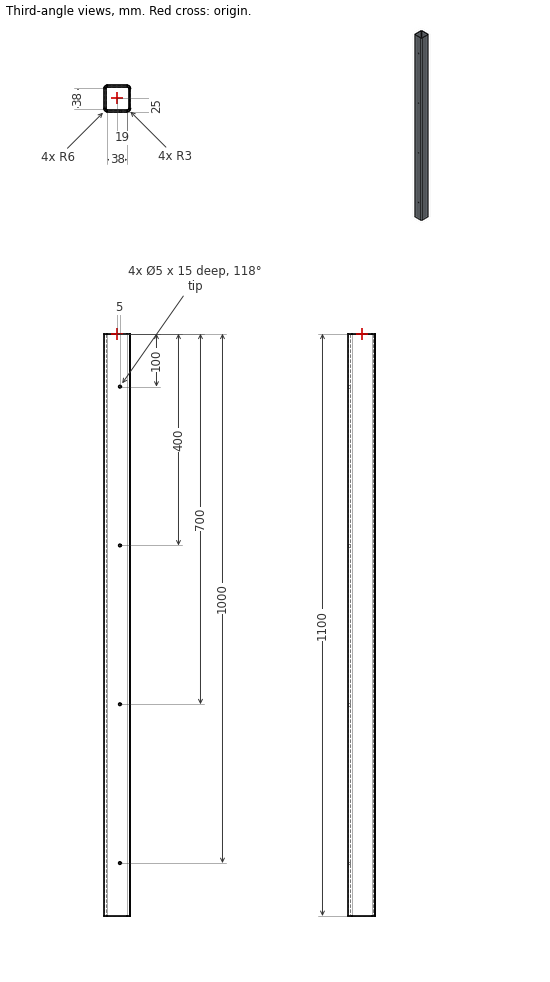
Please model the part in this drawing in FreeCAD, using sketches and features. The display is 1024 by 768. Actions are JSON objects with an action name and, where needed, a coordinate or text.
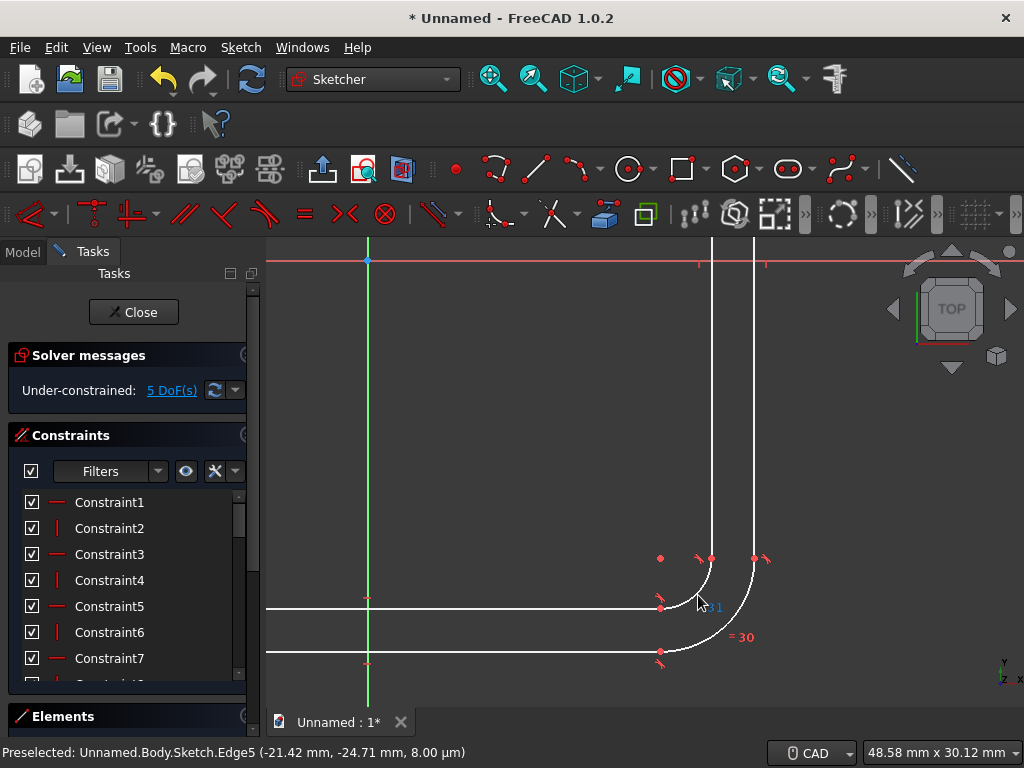
{"action": "left_click", "coordinate": [697, 594]}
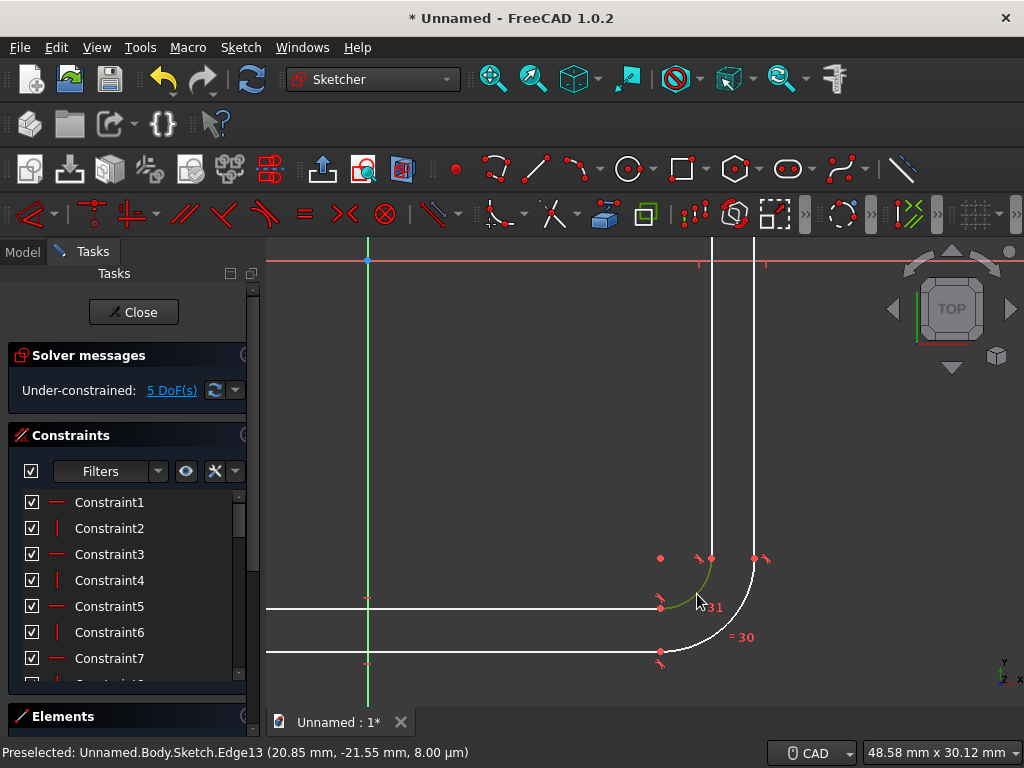
{"action": "key", "text": "k r"}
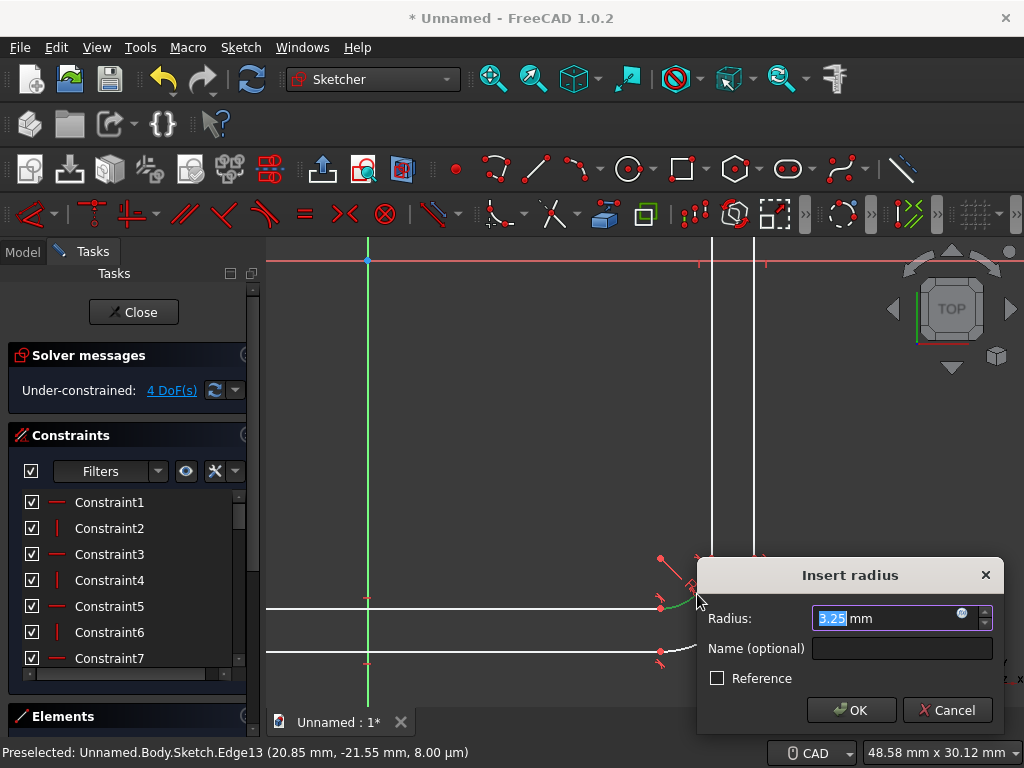
{"action": "type", "text": "3"}
{"action": "key", "text": "Return"}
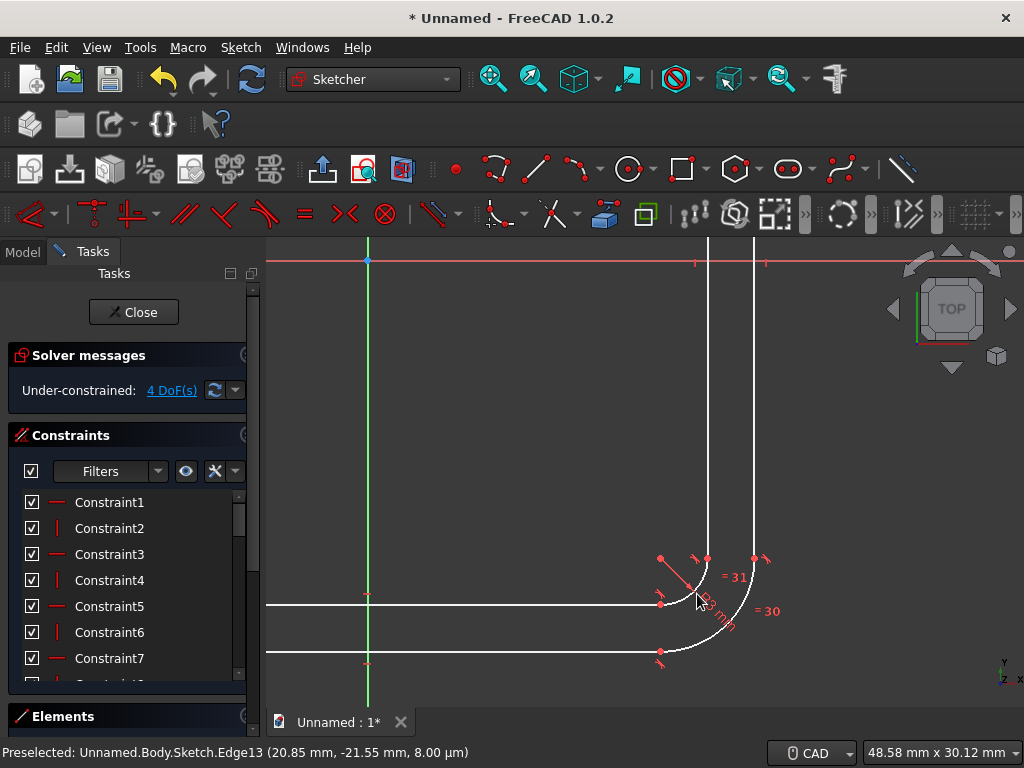
{"action": "left_click", "coordinate": [485, 652]}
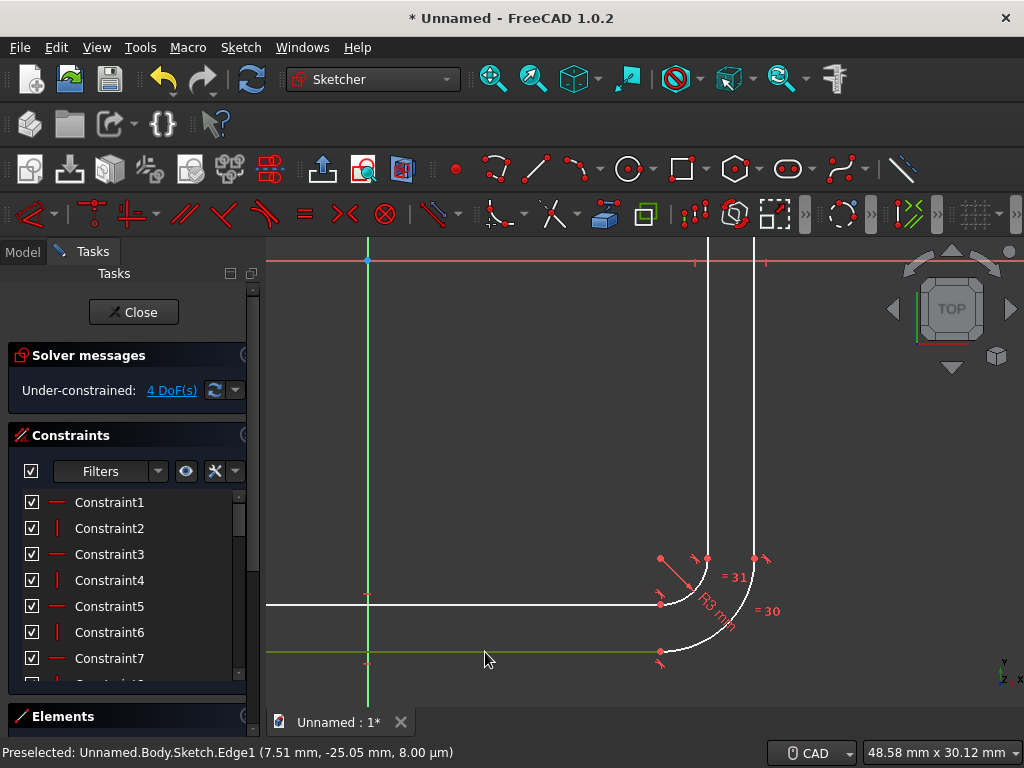
{"action": "key", "text": "l"}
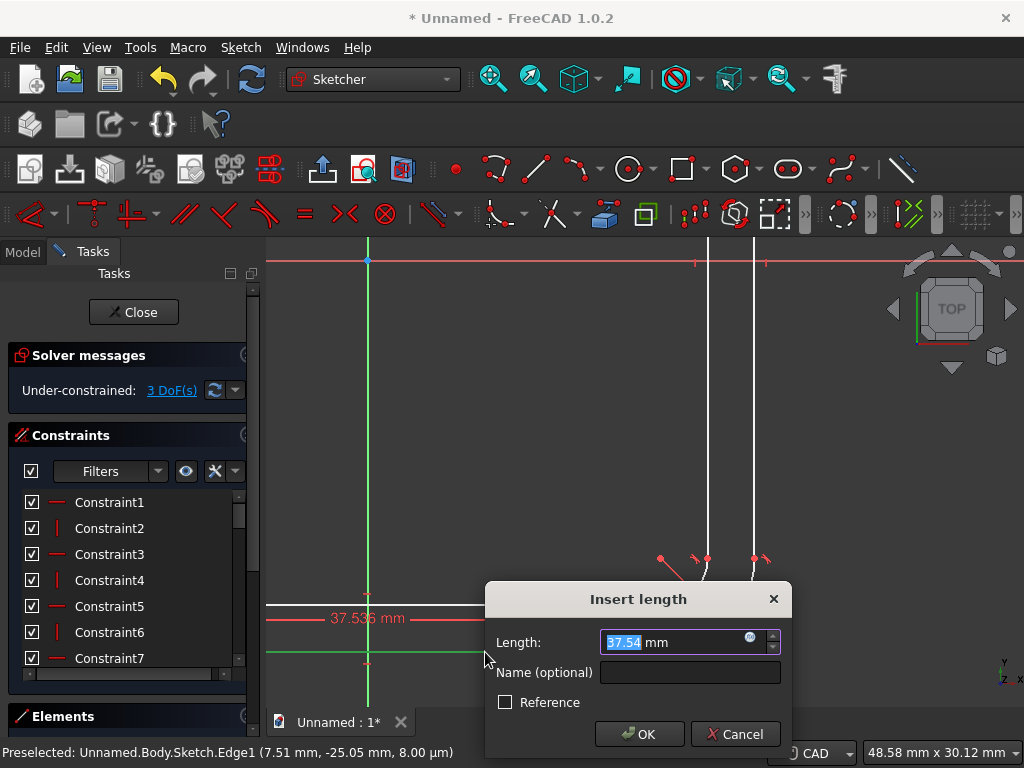
{"action": "type", "text": "38"}
{"action": "key", "text": "Return"}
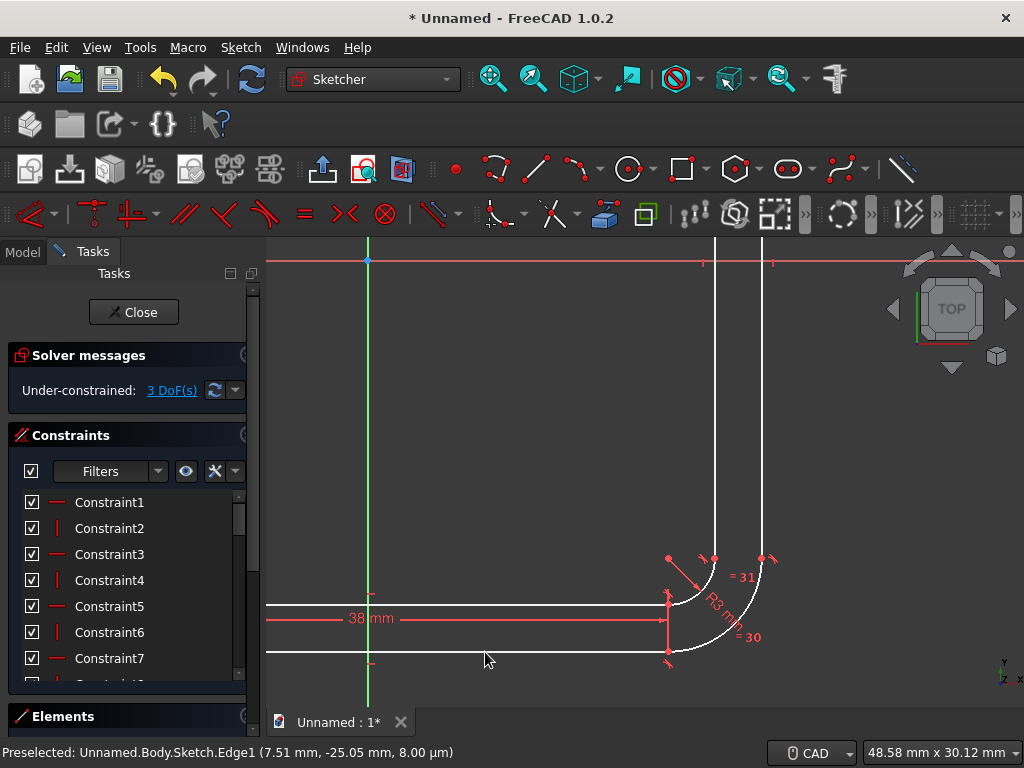
{"action": "scroll", "coordinate": [698, 595], "scroll_direction": "down", "scroll_amount": 5}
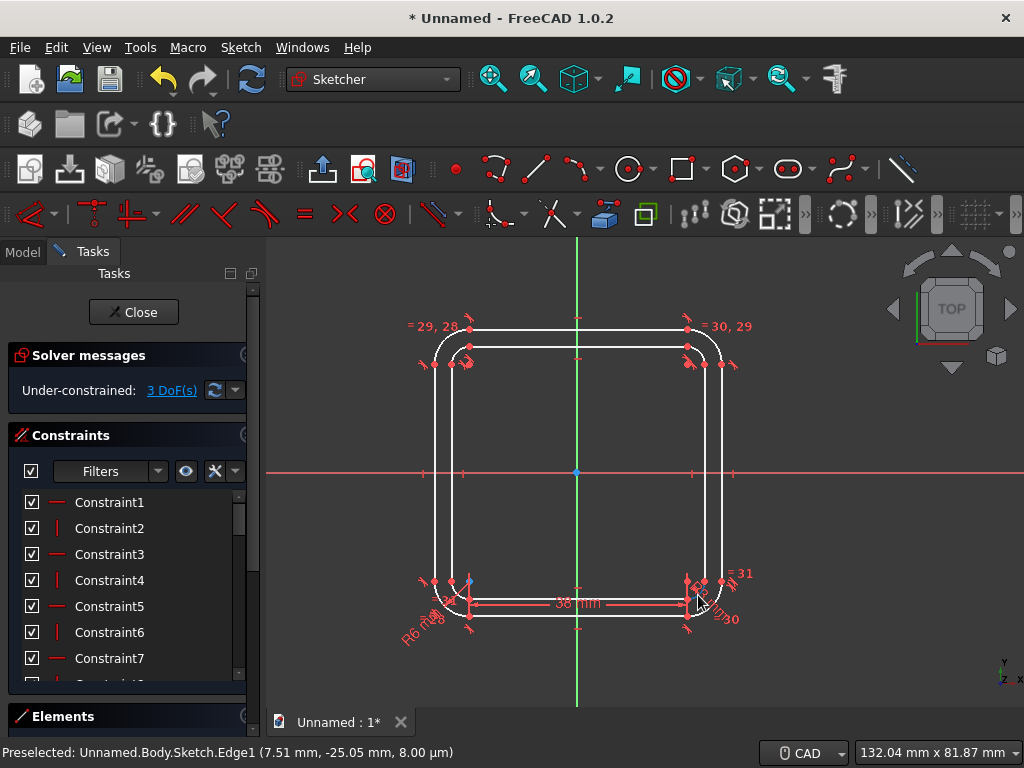
{"action": "left_click", "coordinate": [435, 517]}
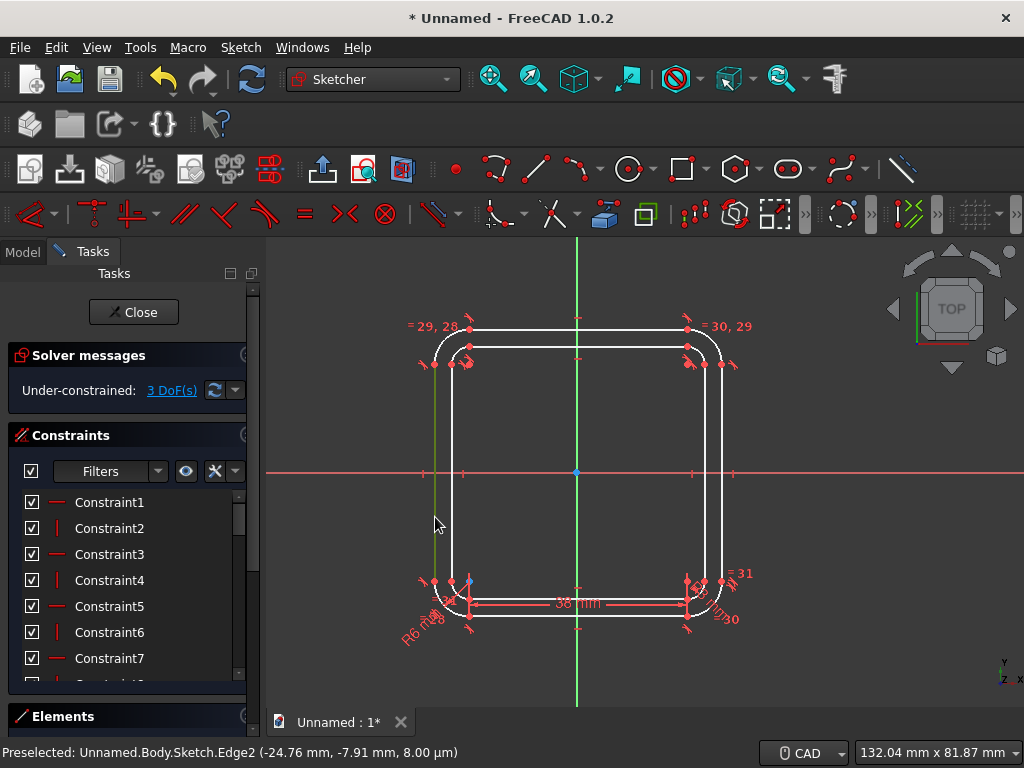
{"action": "key", "text": "i"}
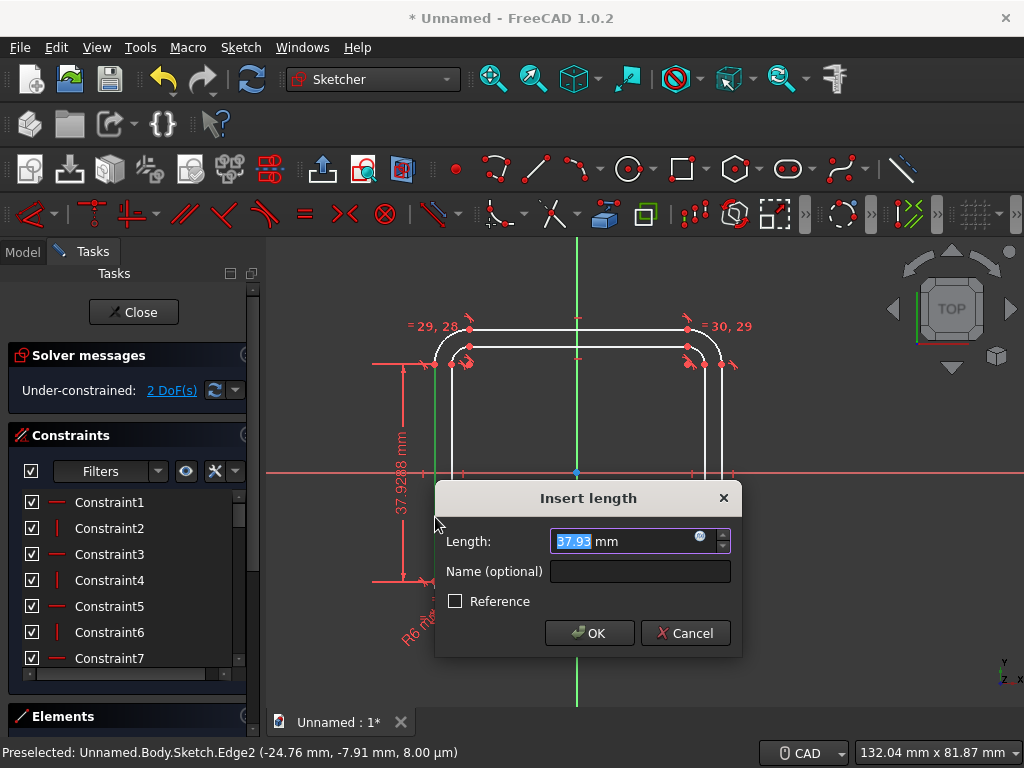
{"action": "type", "text": "38"}
{"action": "key", "text": "Return"}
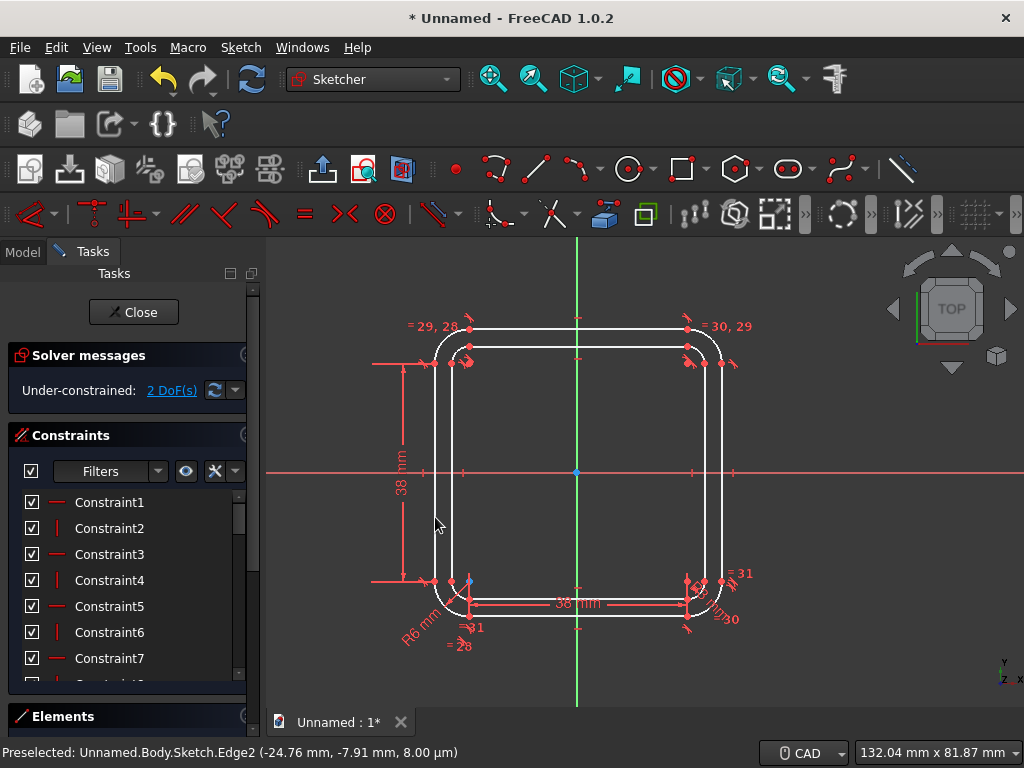
{"action": "left_click", "coordinate": [687, 616]}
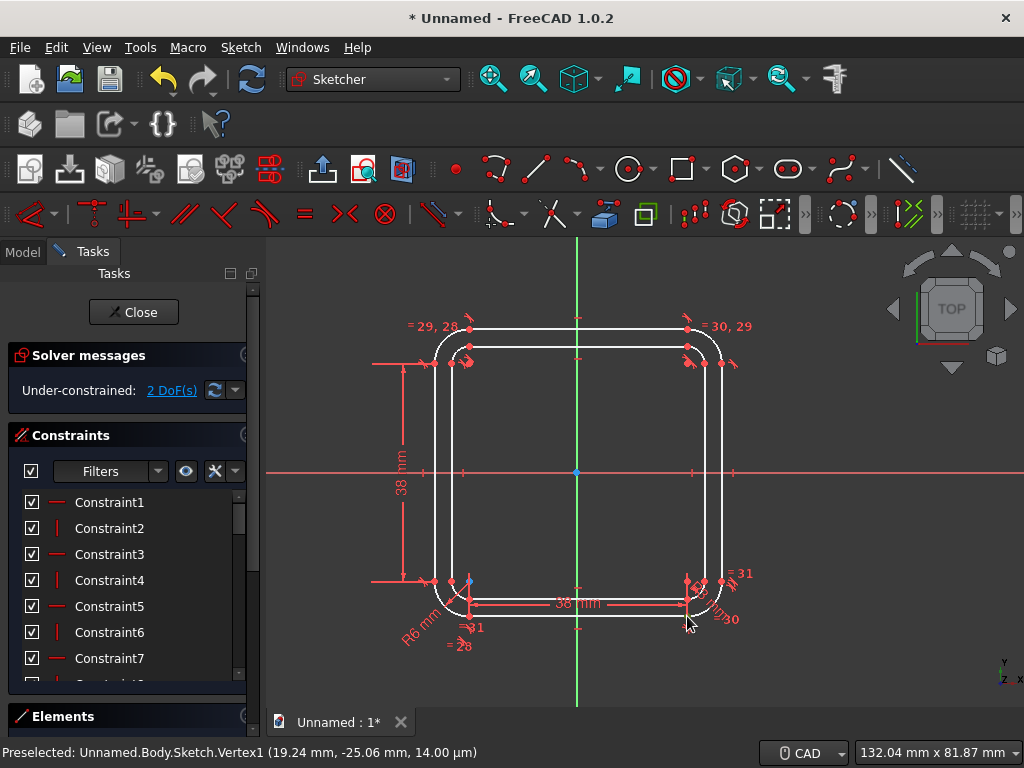
{"action": "key", "text": "l"}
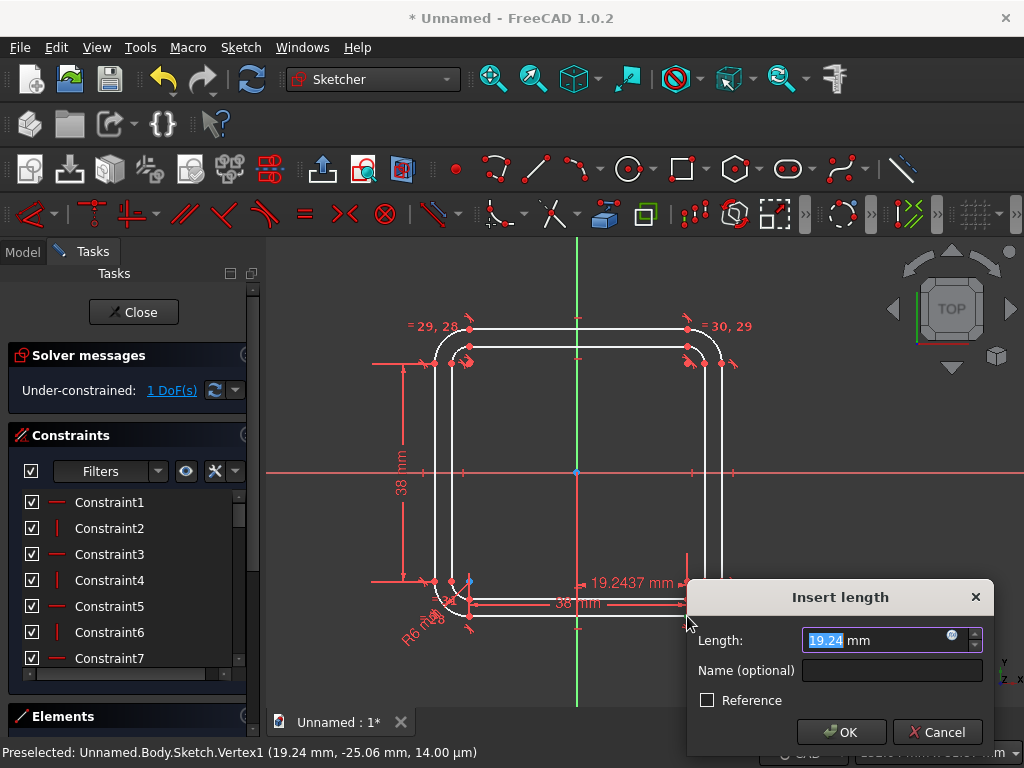
{"action": "type", "text": "19"}
{"action": "key", "text": "Return"}